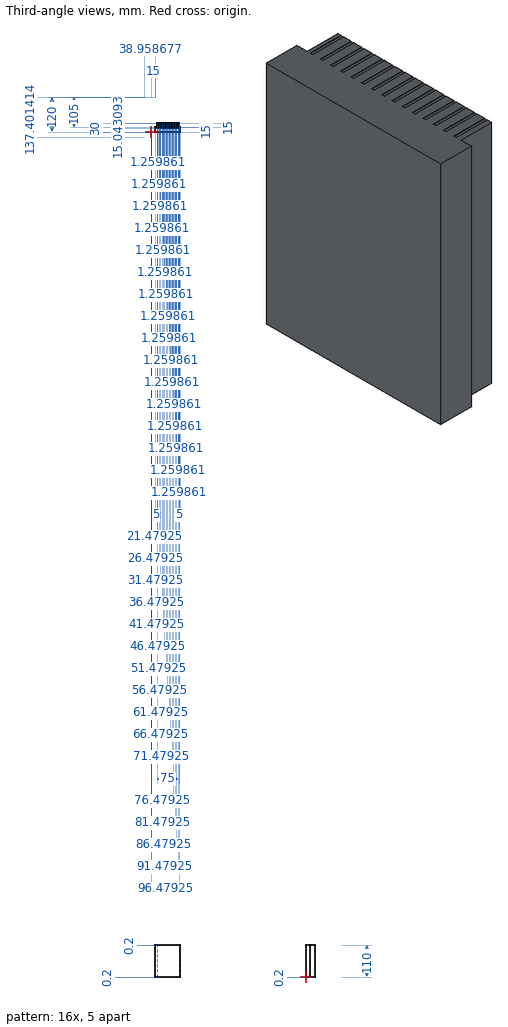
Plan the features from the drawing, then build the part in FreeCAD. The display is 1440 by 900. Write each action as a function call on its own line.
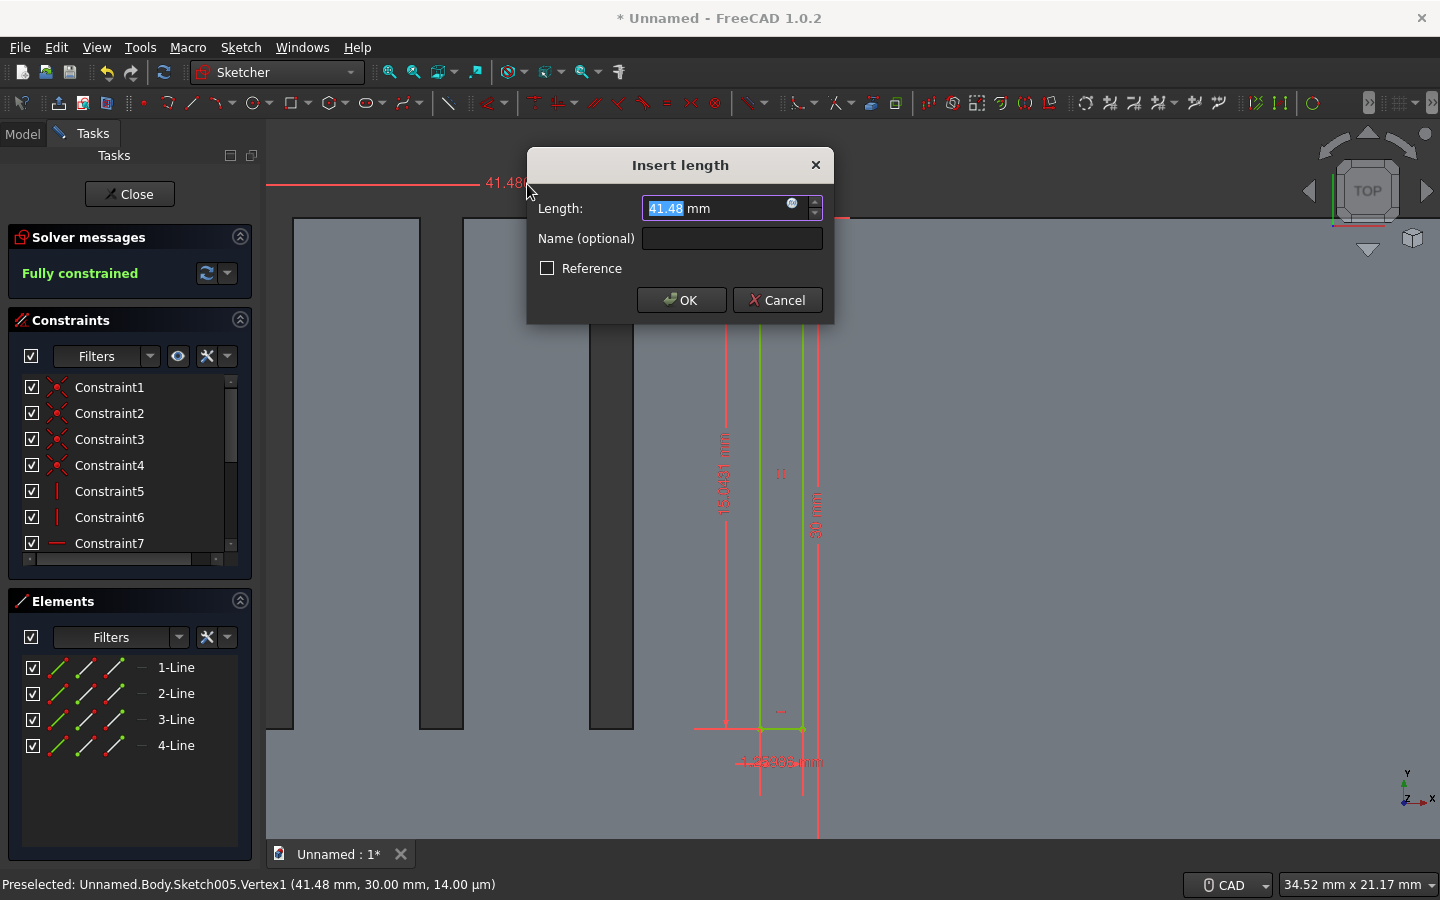
text(41.47925)
key(Return)
key(Escape)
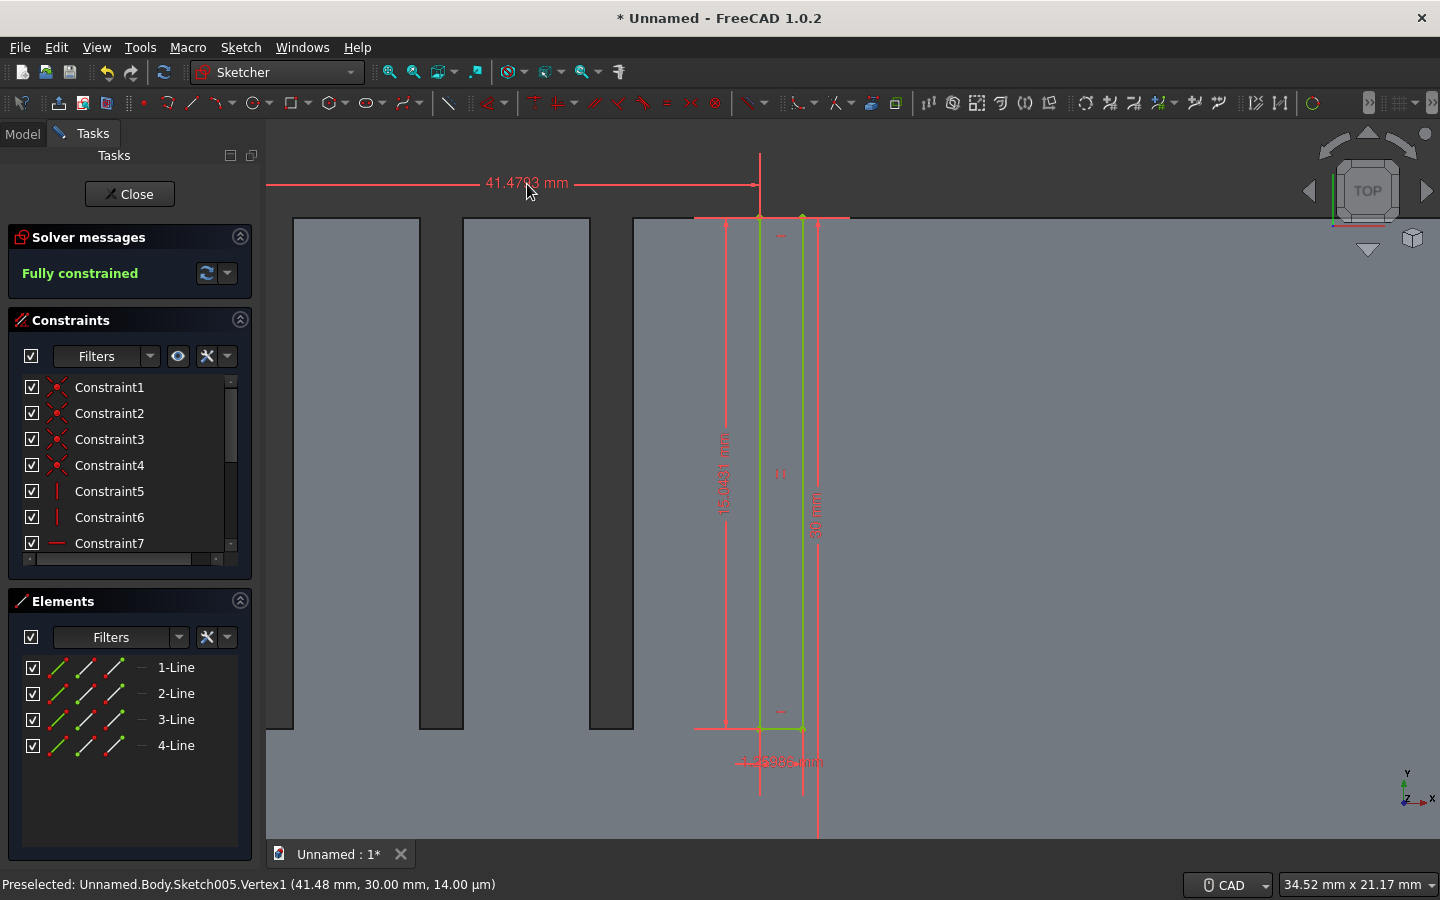
click(130, 194)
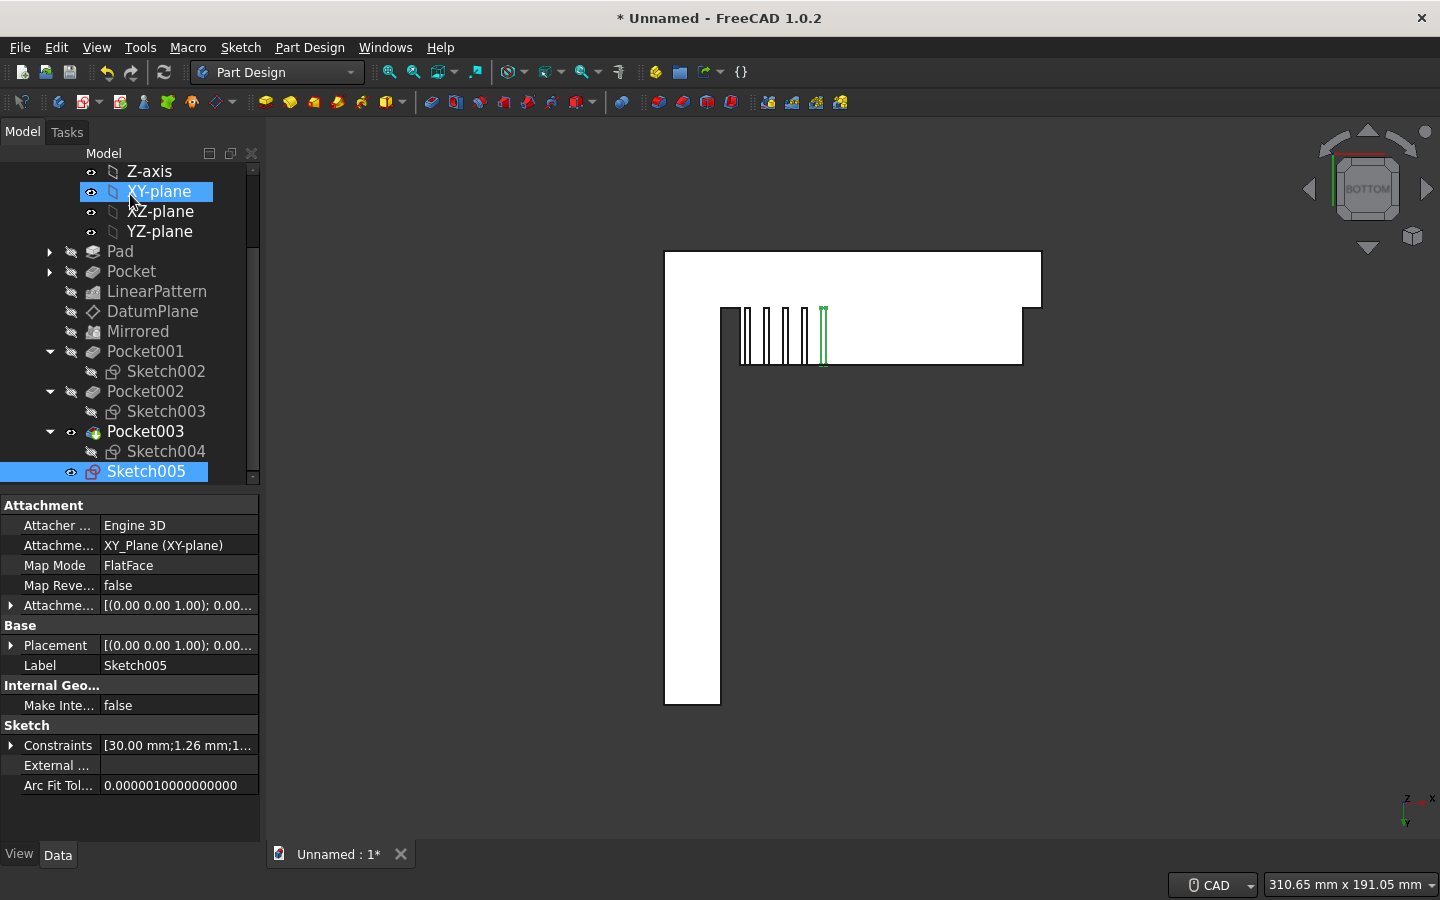
click(432, 102)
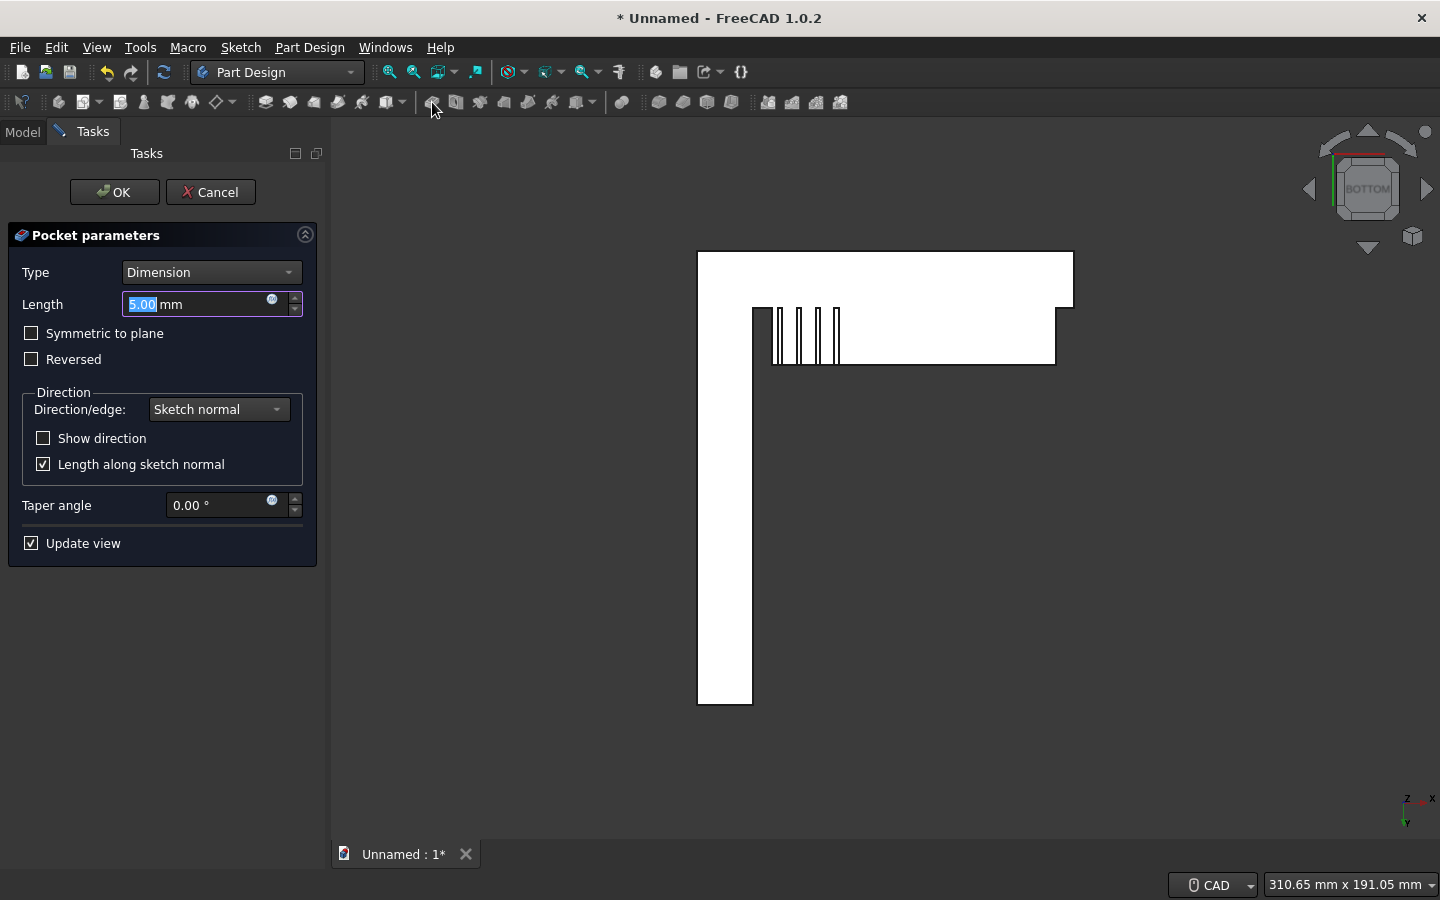
text(0.2)
key(Tab)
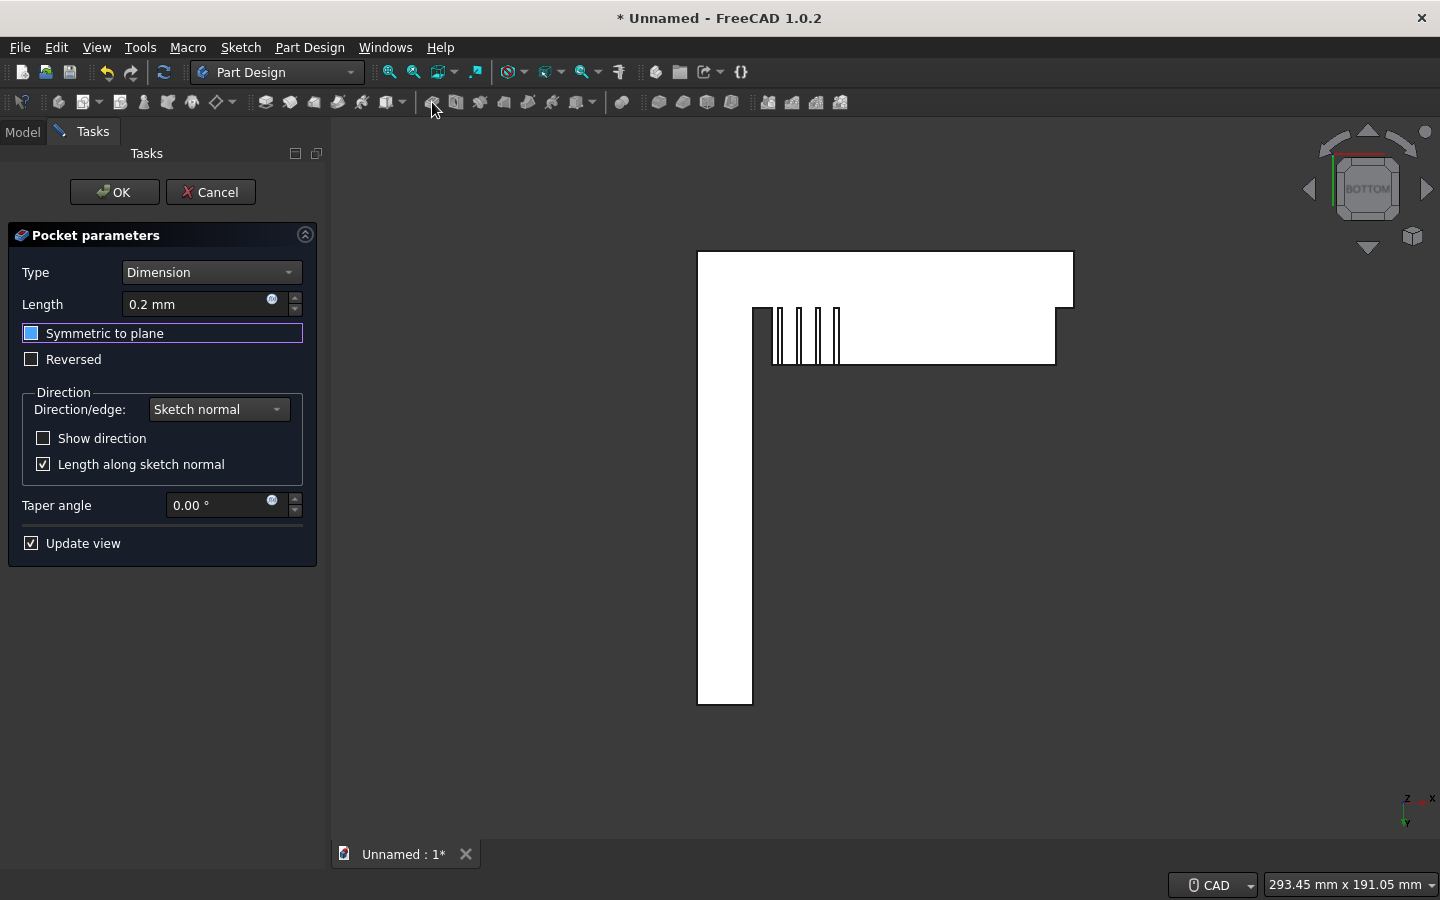
click(30, 359)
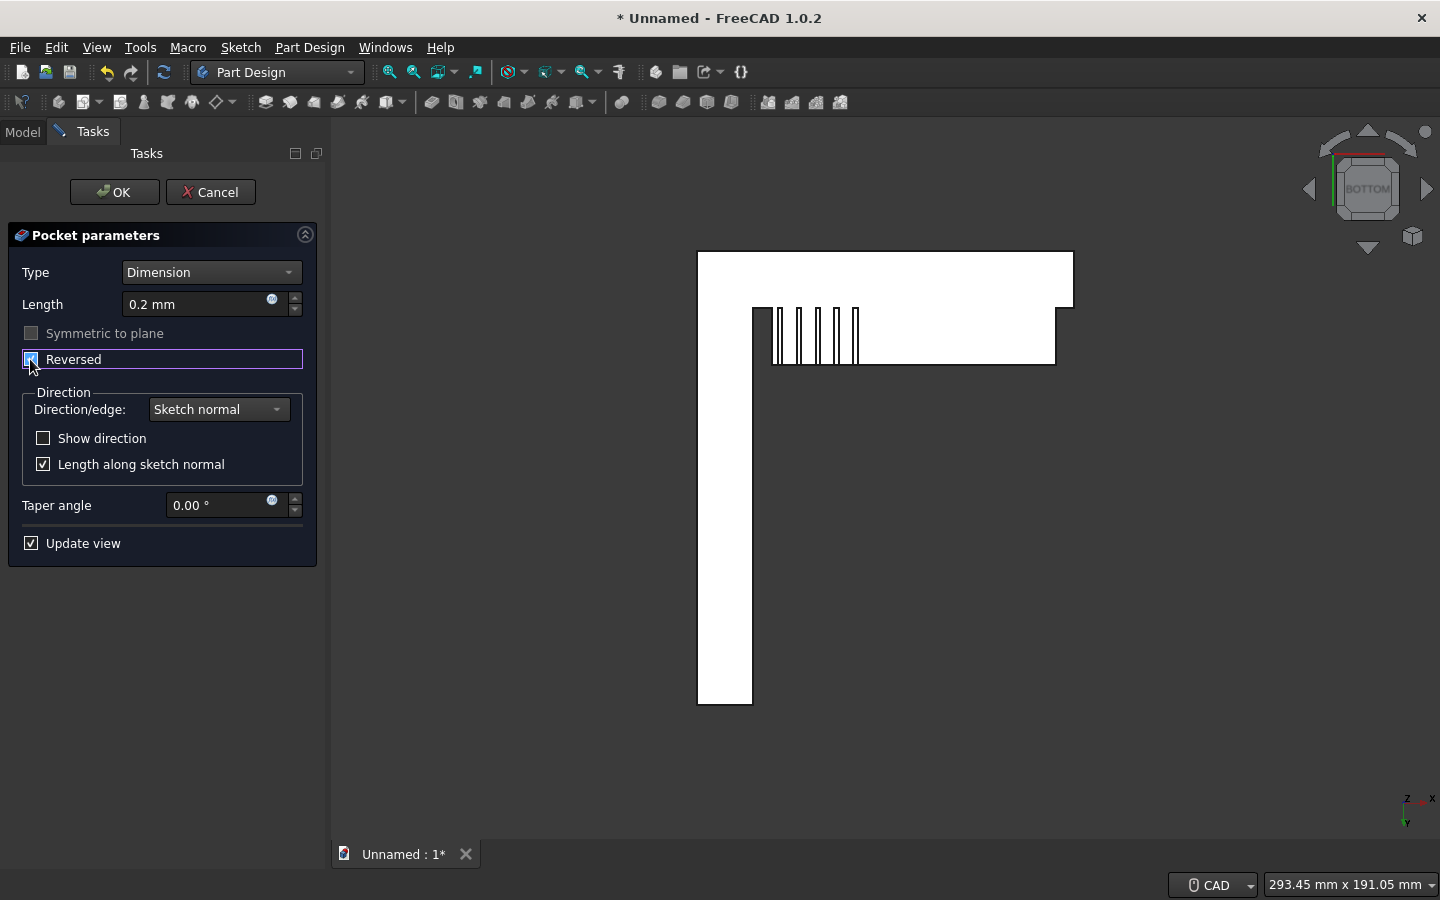
click(115, 192)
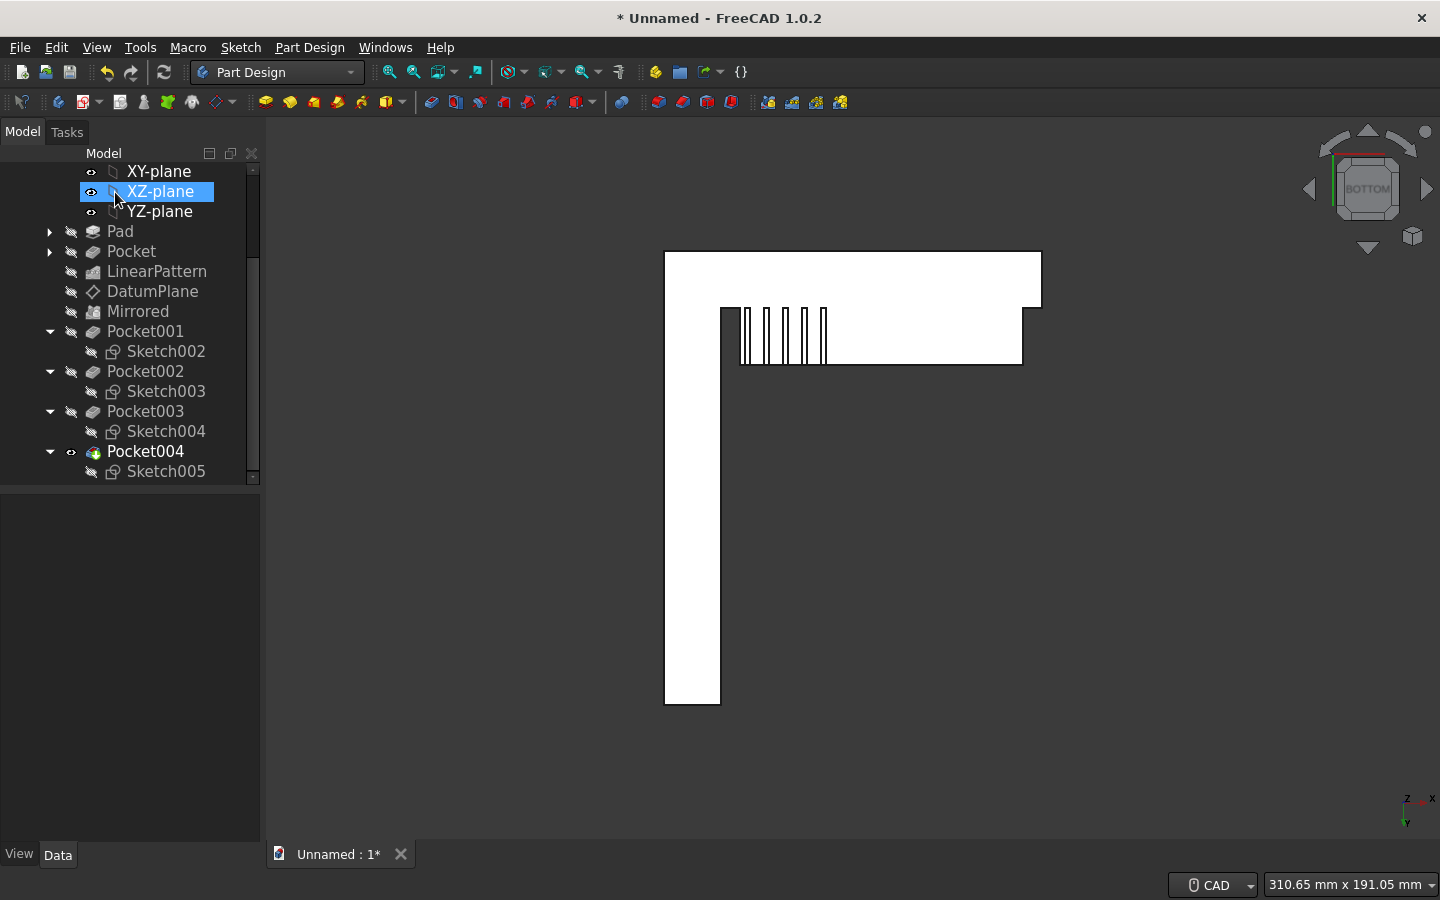
click(84, 102)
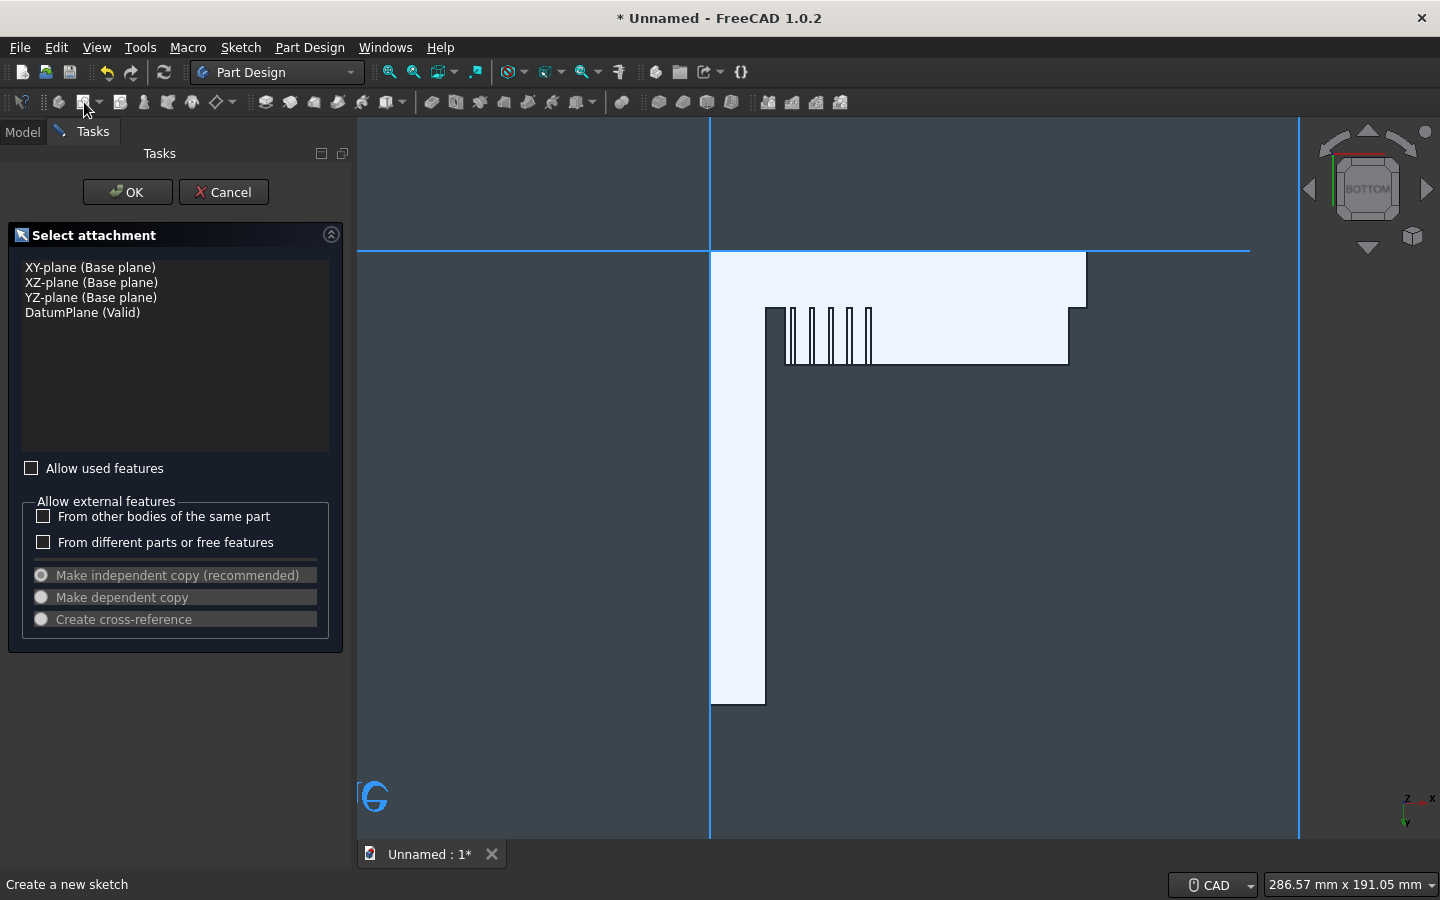
click(82, 268)